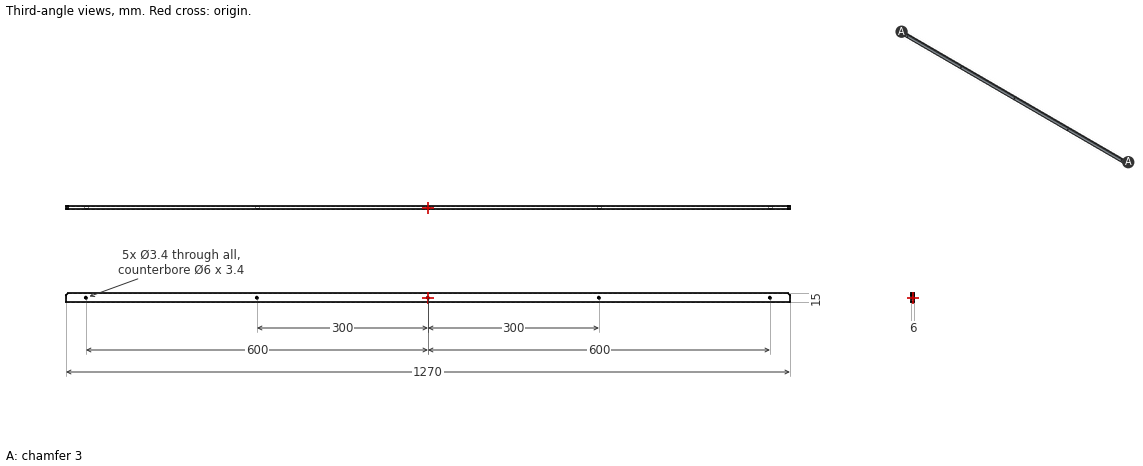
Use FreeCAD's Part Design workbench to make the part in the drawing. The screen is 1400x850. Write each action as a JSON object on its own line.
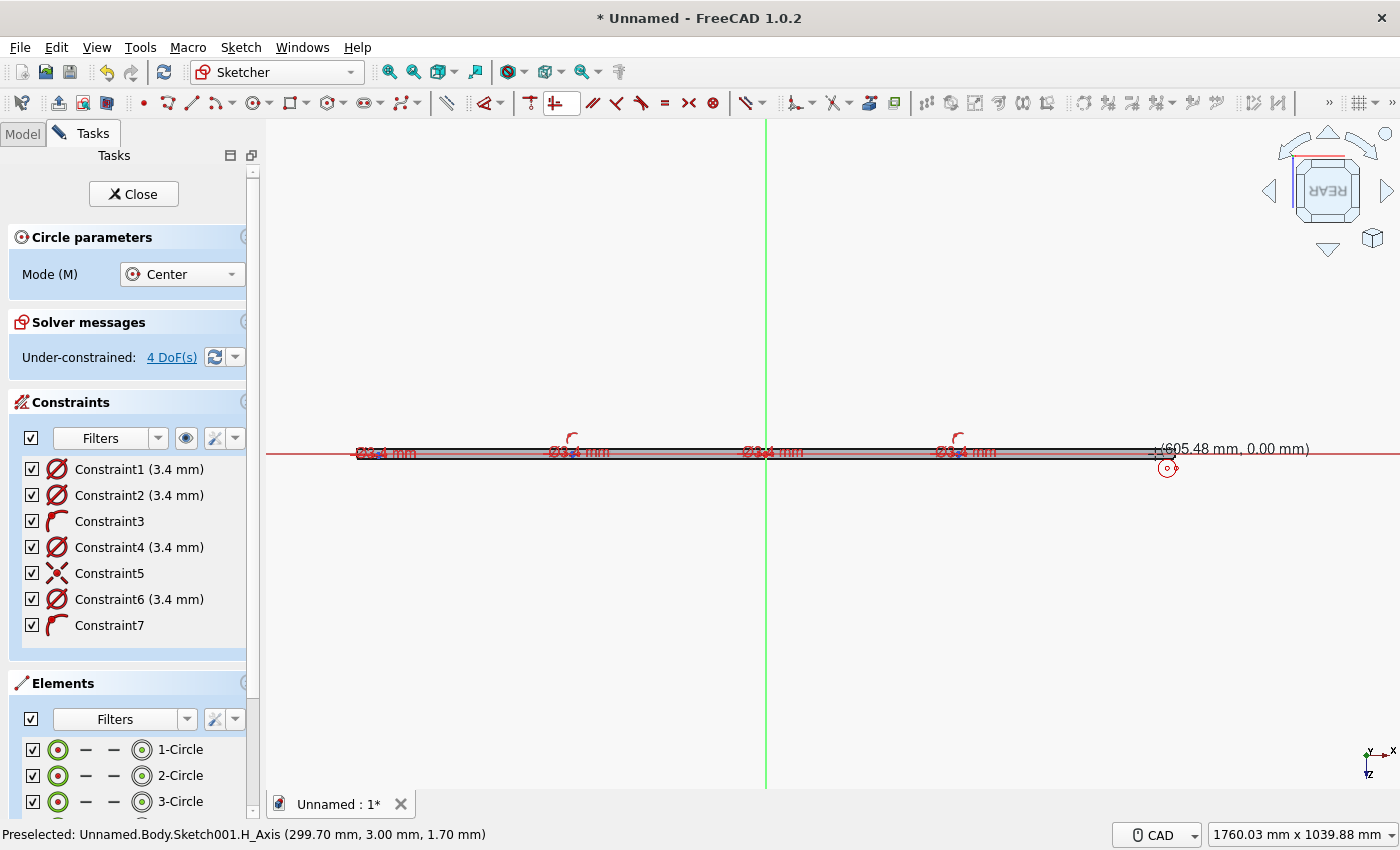
{"action": "left_click", "coordinate": [1152, 454]}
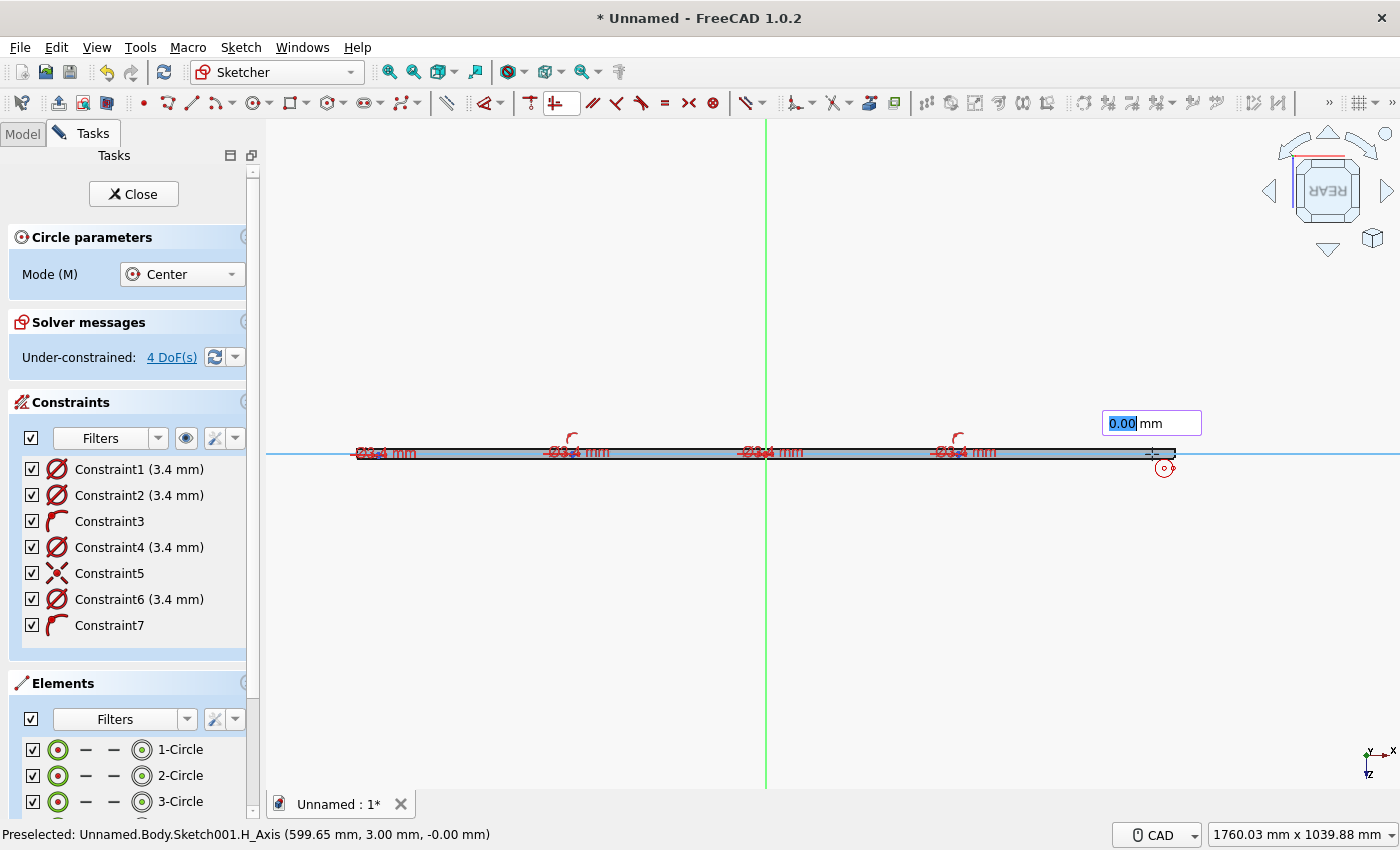
{"action": "scroll", "coordinate": [1152, 455], "scroll_direction": "up", "scroll_amount": 14}
{"action": "mouse_move", "coordinate": [1137, 450]}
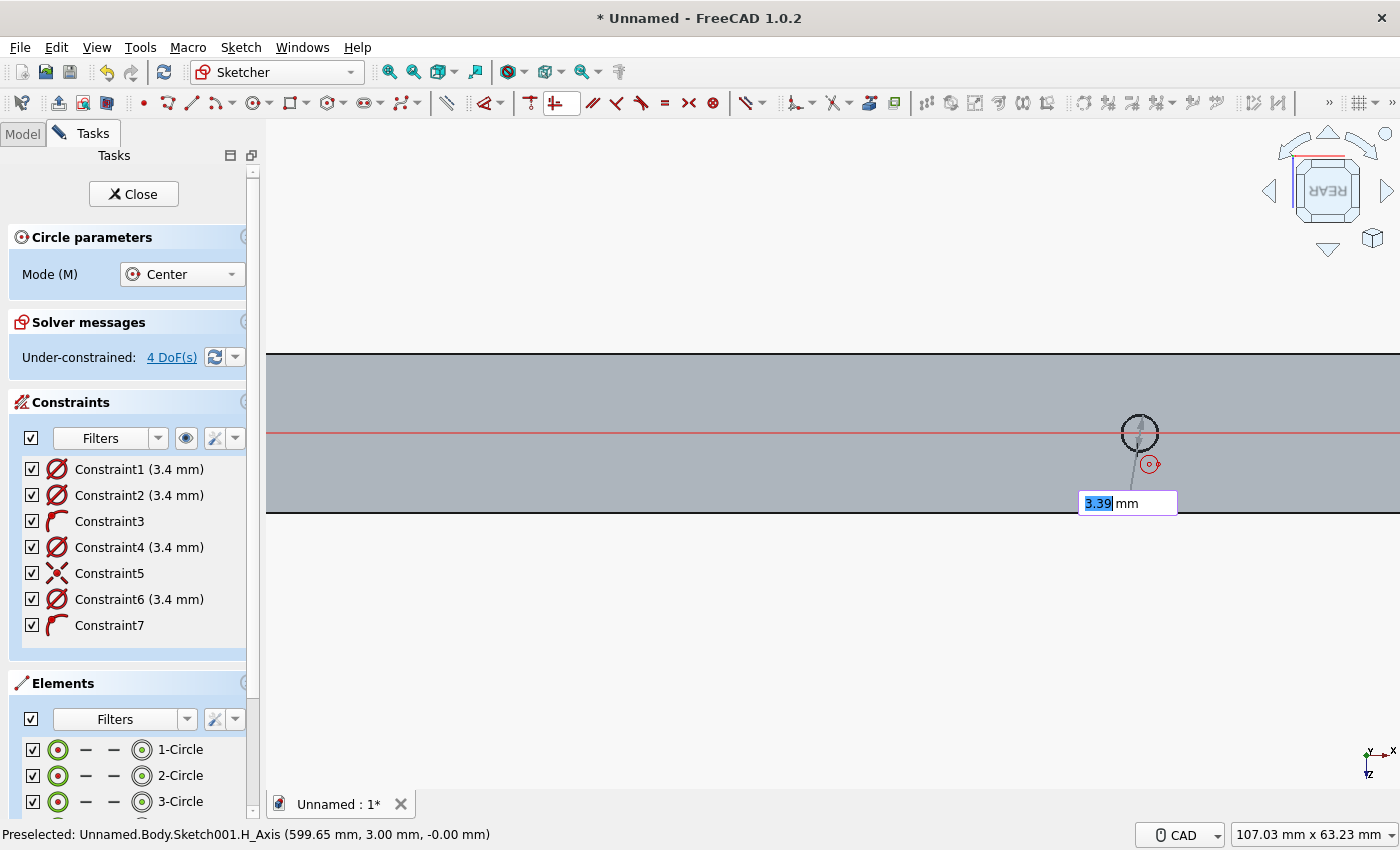
{"action": "type", "text": "3.4"}
{"action": "key", "text": "Return"}
{"action": "key", "text": "Escape"}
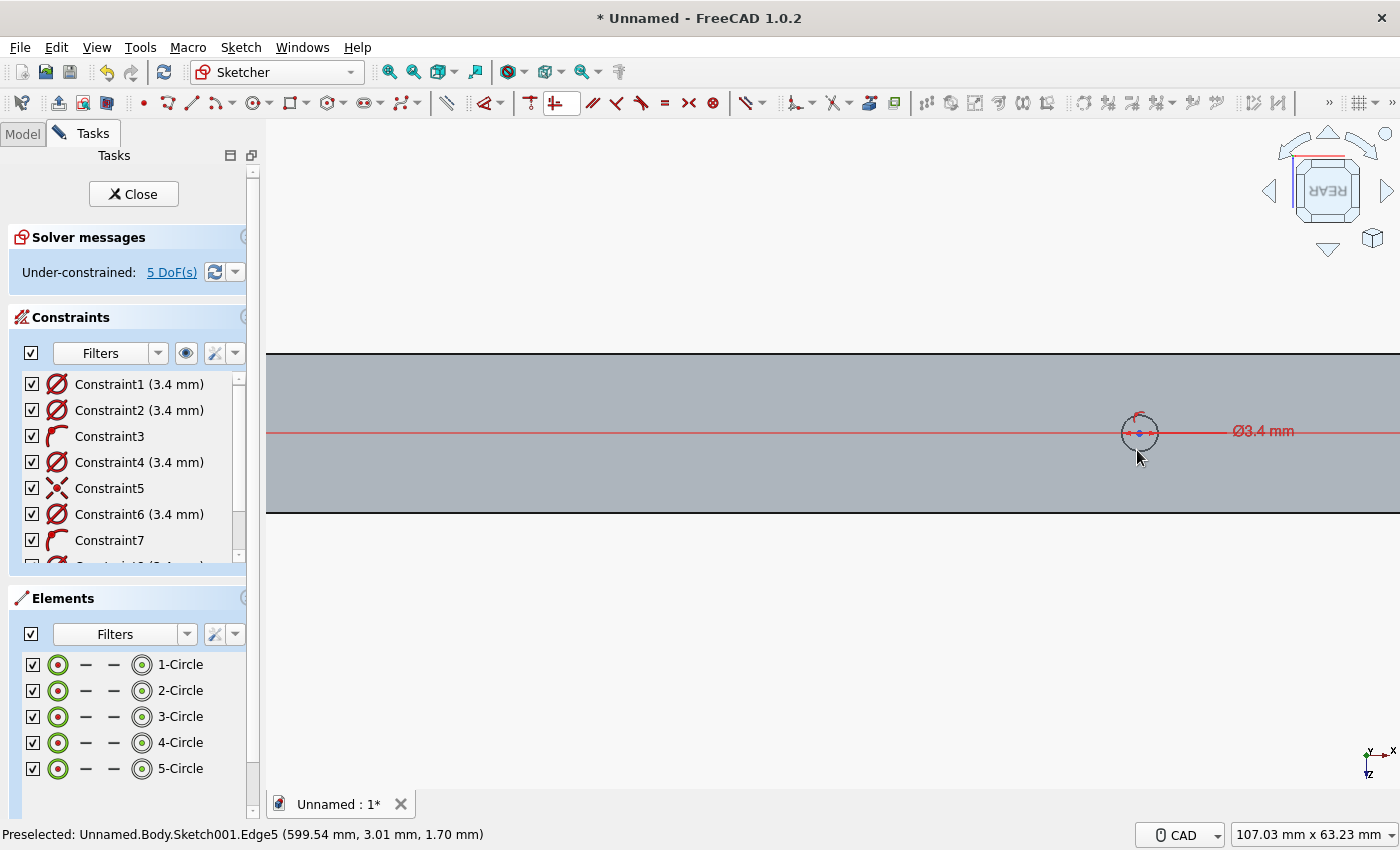
{"action": "scroll", "coordinate": [1078, 455], "scroll_direction": "down", "scroll_amount": 15}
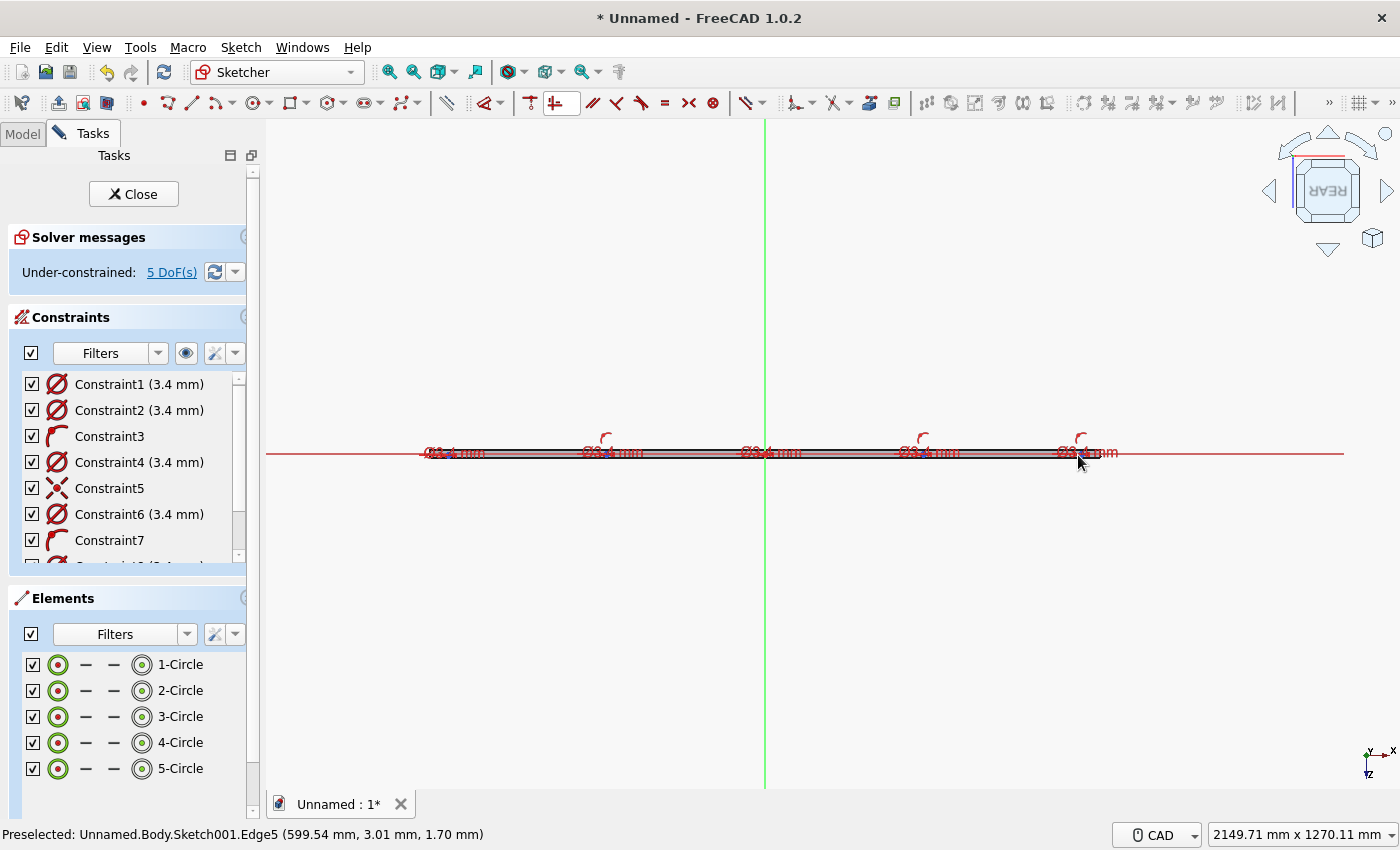
{"action": "left_click", "coordinate": [449, 455]}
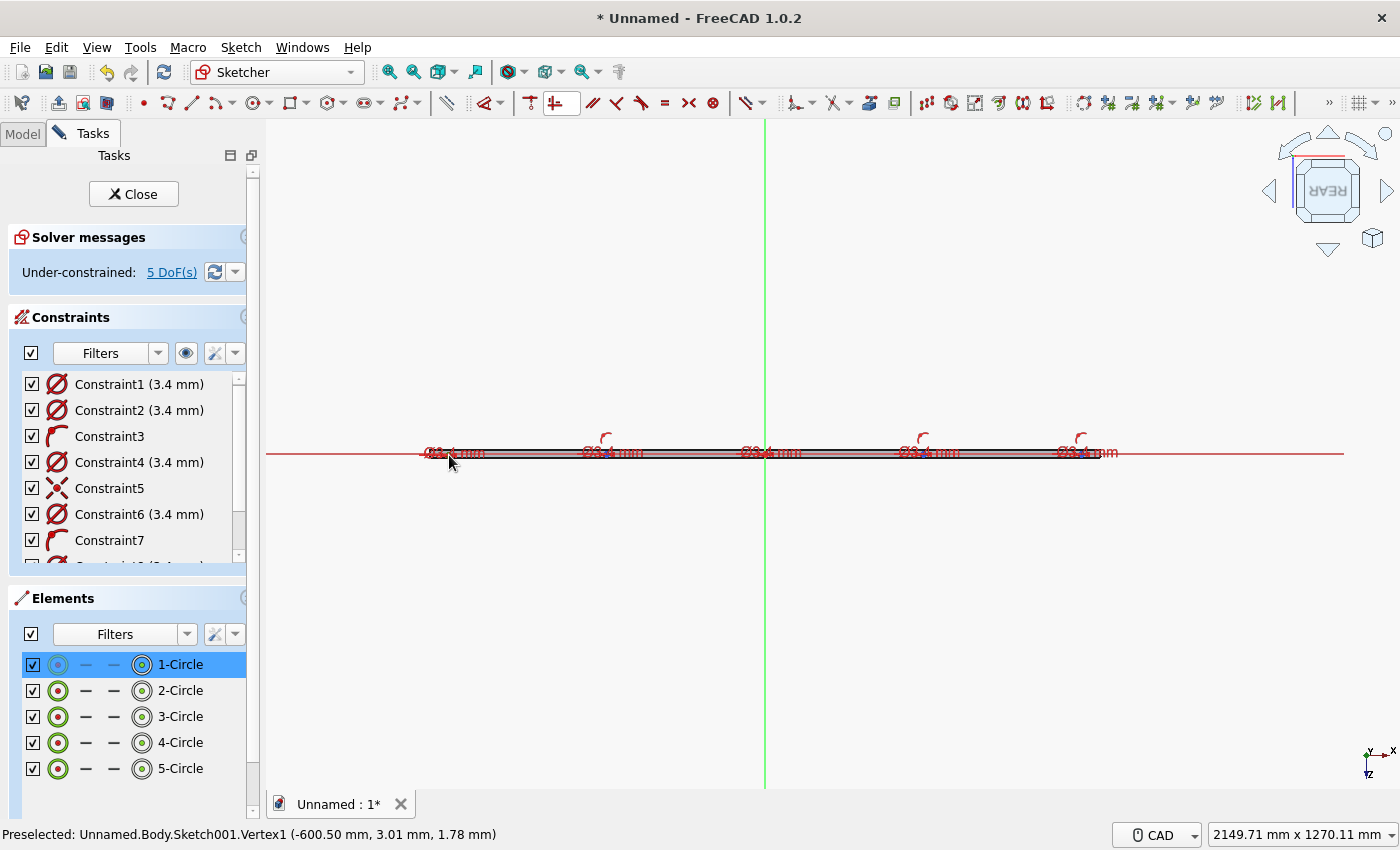
{"action": "left_click", "coordinate": [361, 454]}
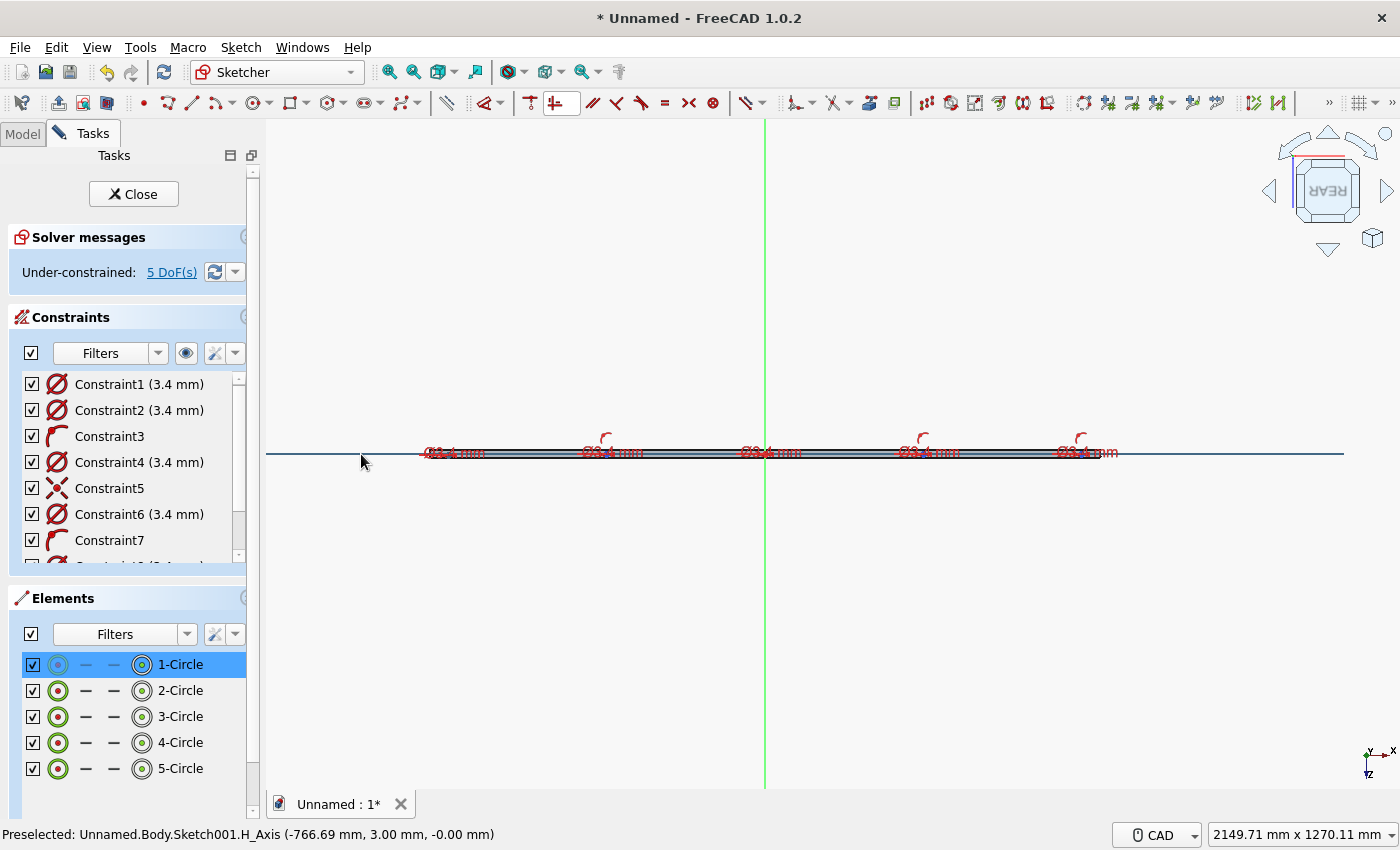
{"action": "key", "text": "c"}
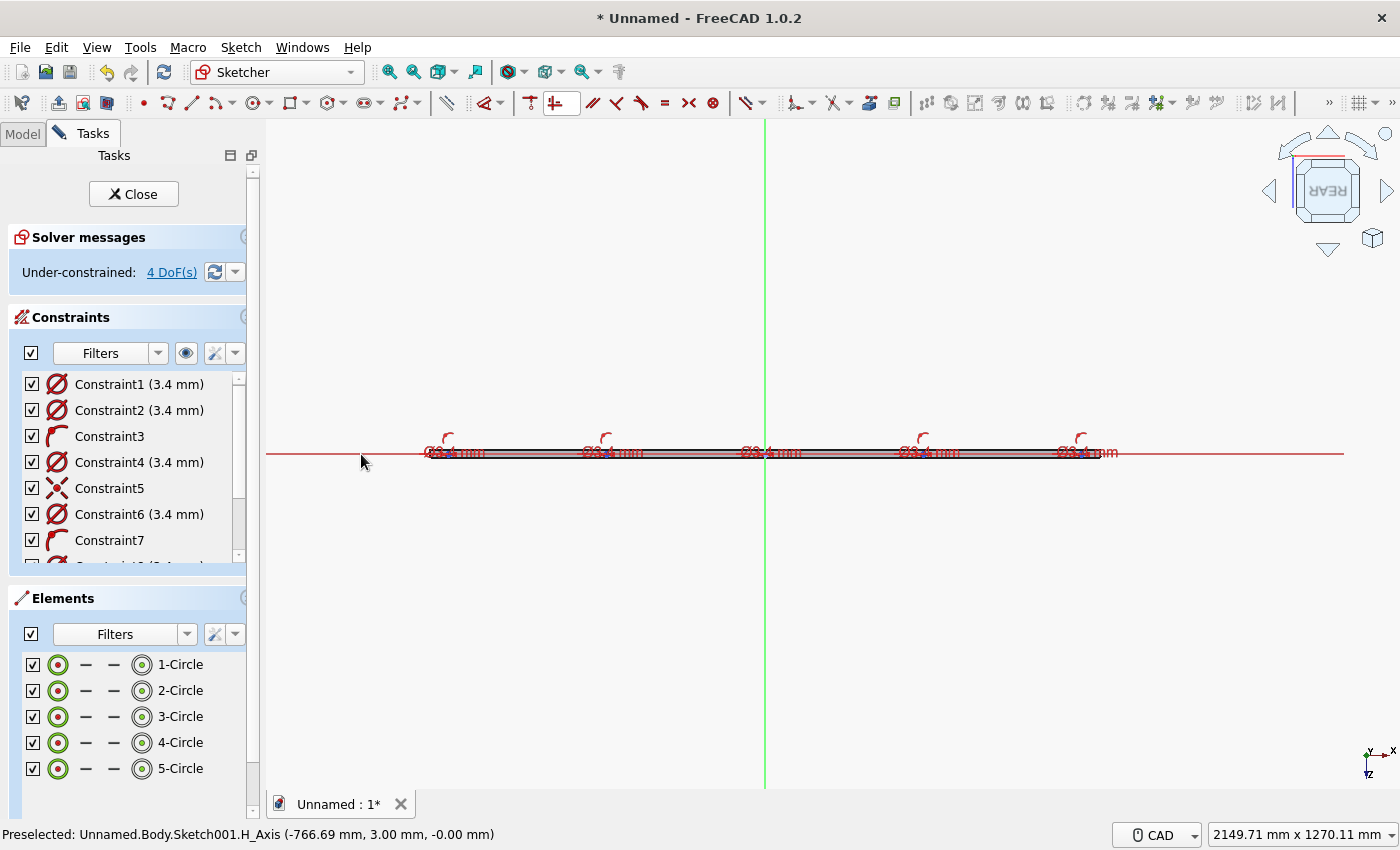
{"action": "left_click", "coordinate": [484, 104]}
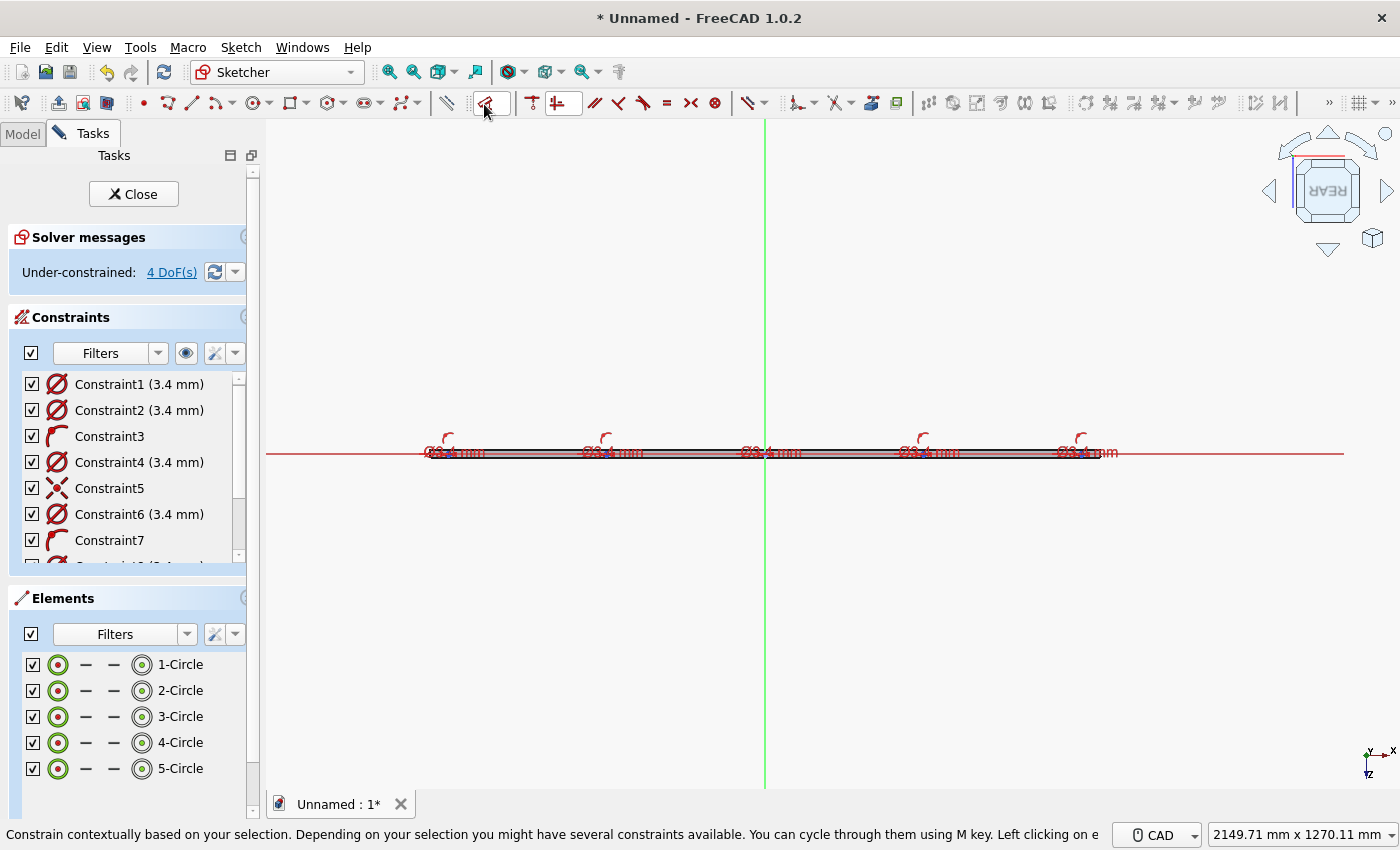
{"action": "left_click", "coordinate": [449, 454]}
{"action": "left_click", "coordinate": [607, 488]}